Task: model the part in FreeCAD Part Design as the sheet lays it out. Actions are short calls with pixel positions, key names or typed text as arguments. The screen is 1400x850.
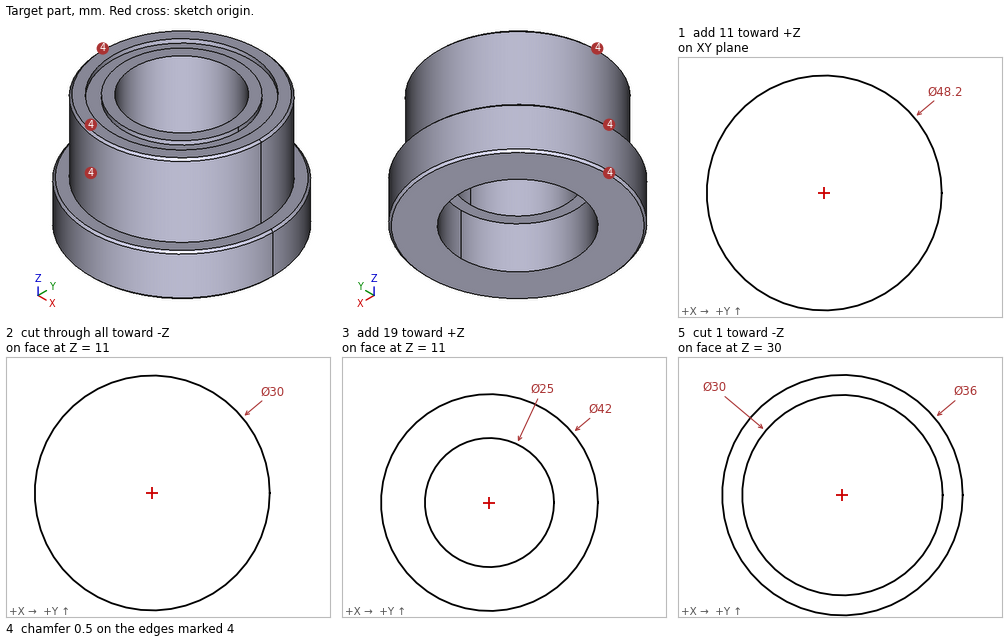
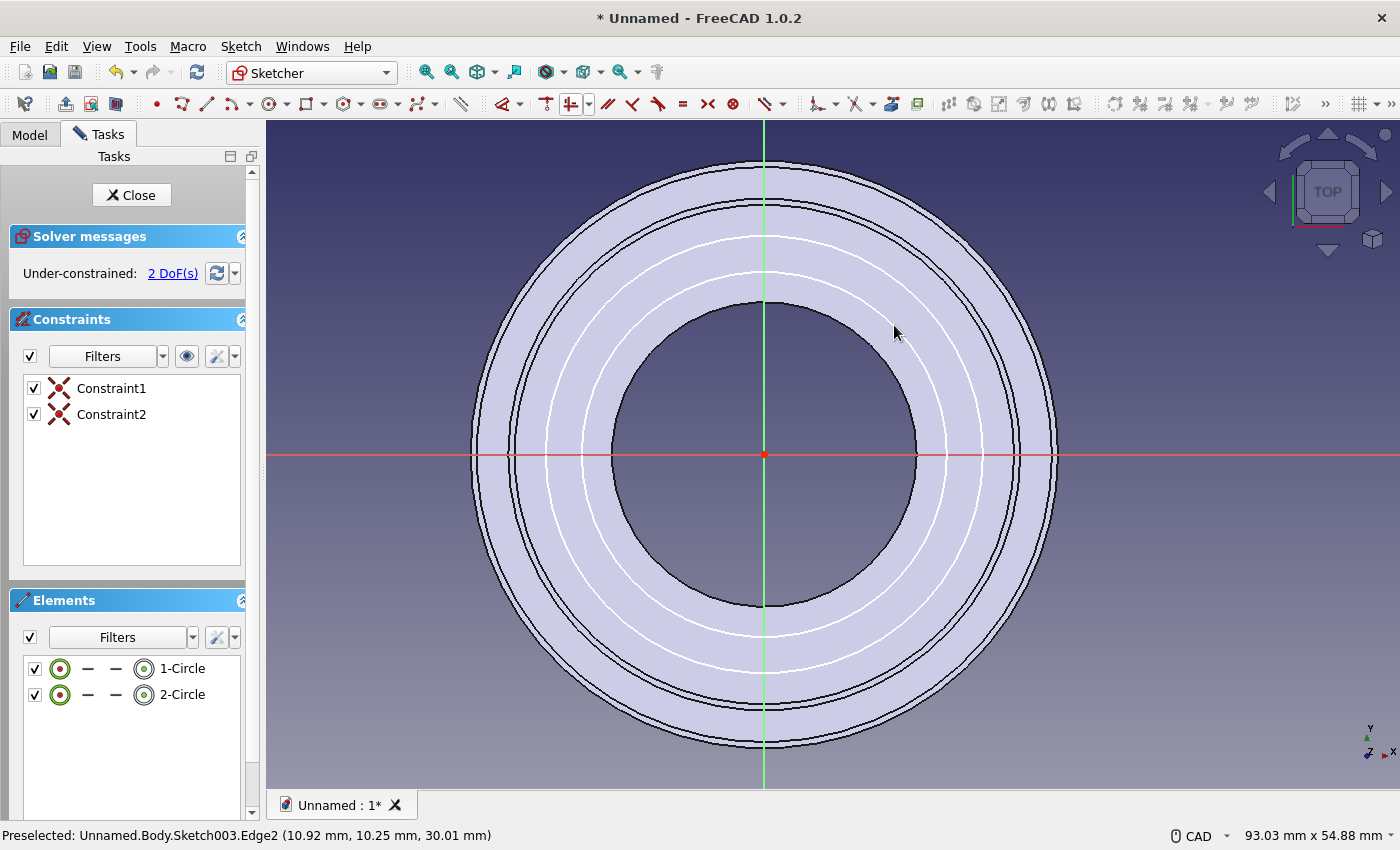
key(d)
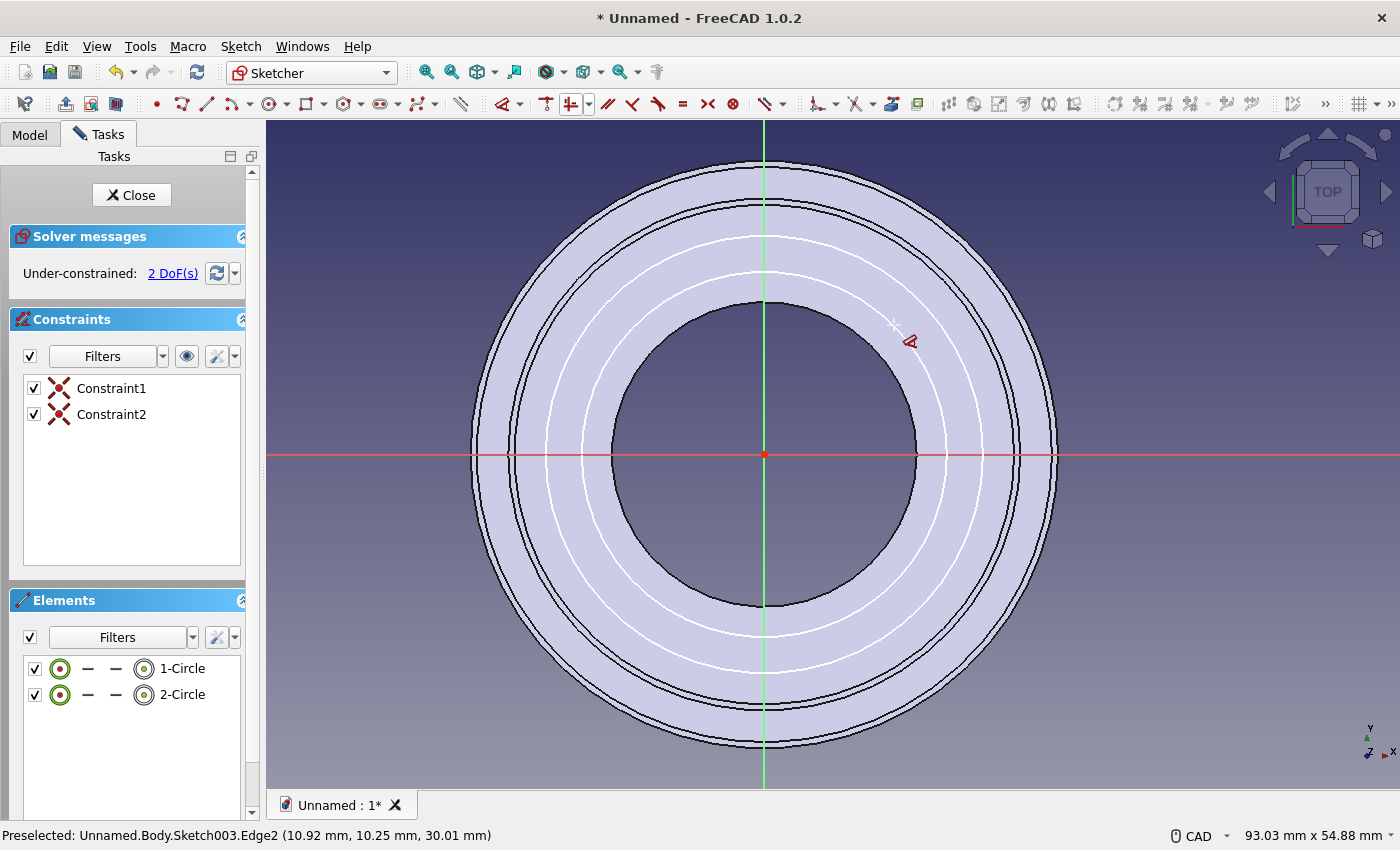
click(918, 299)
click(940, 276)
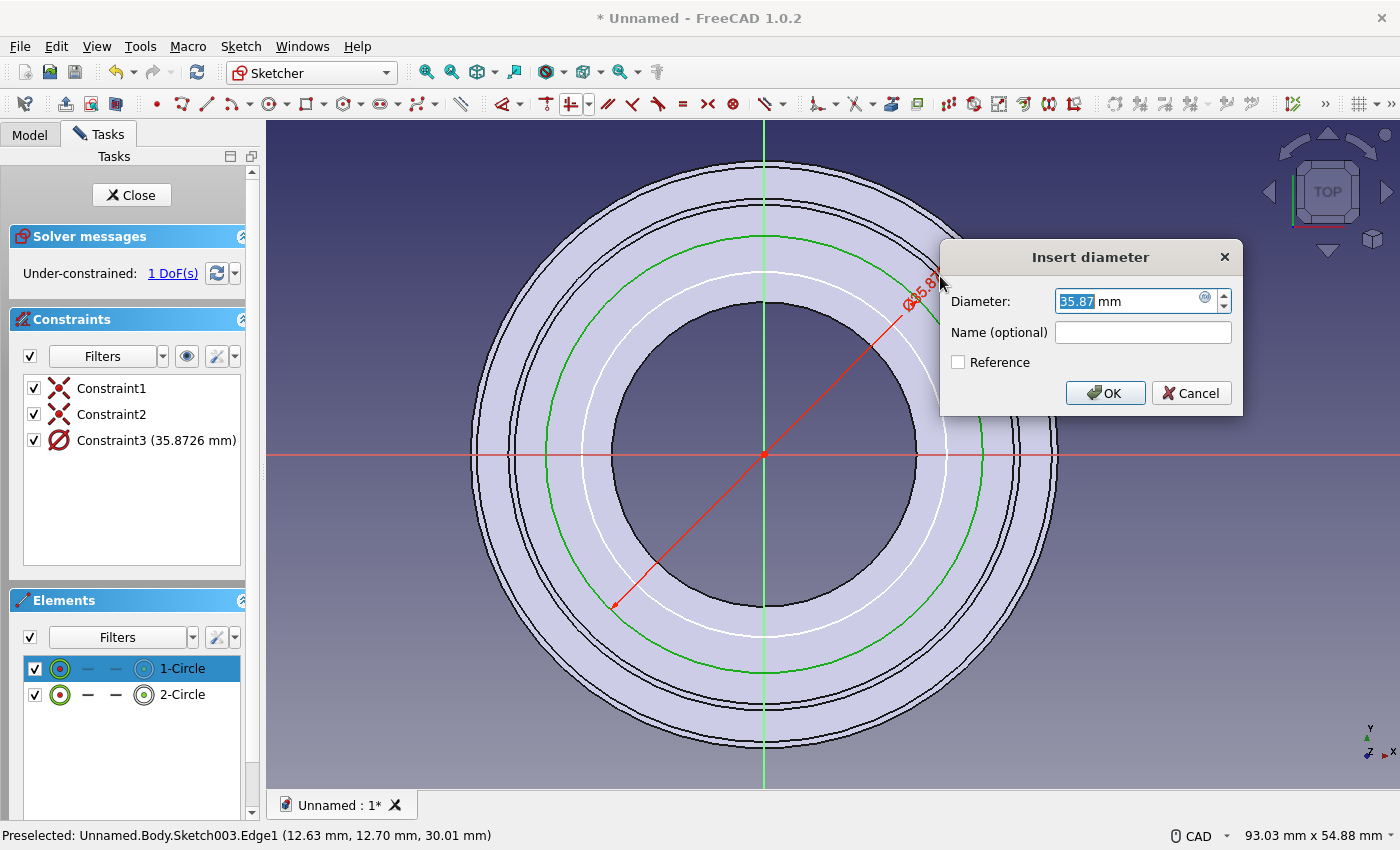
text(36)
key(Return)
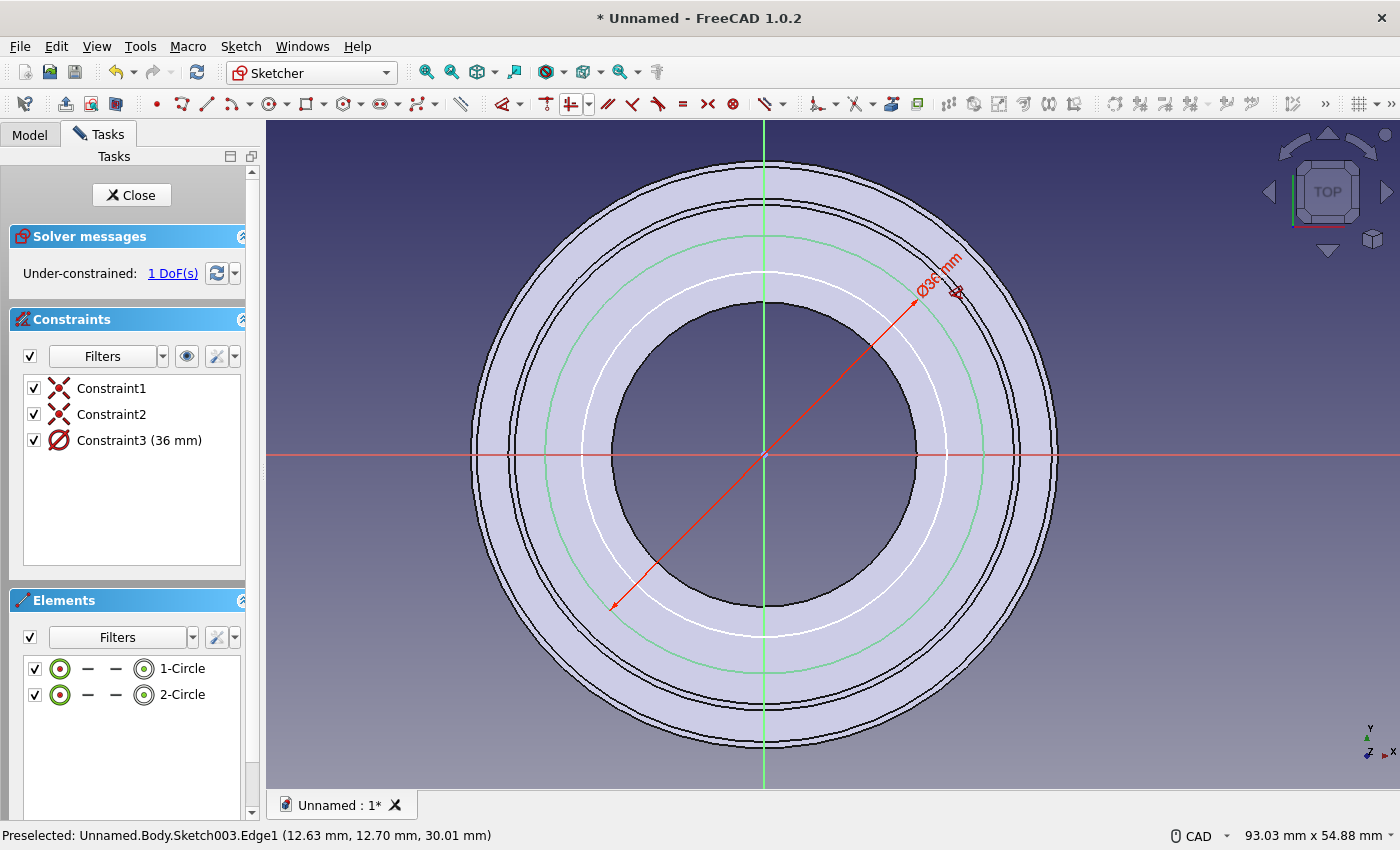
click(893, 325)
click(992, 387)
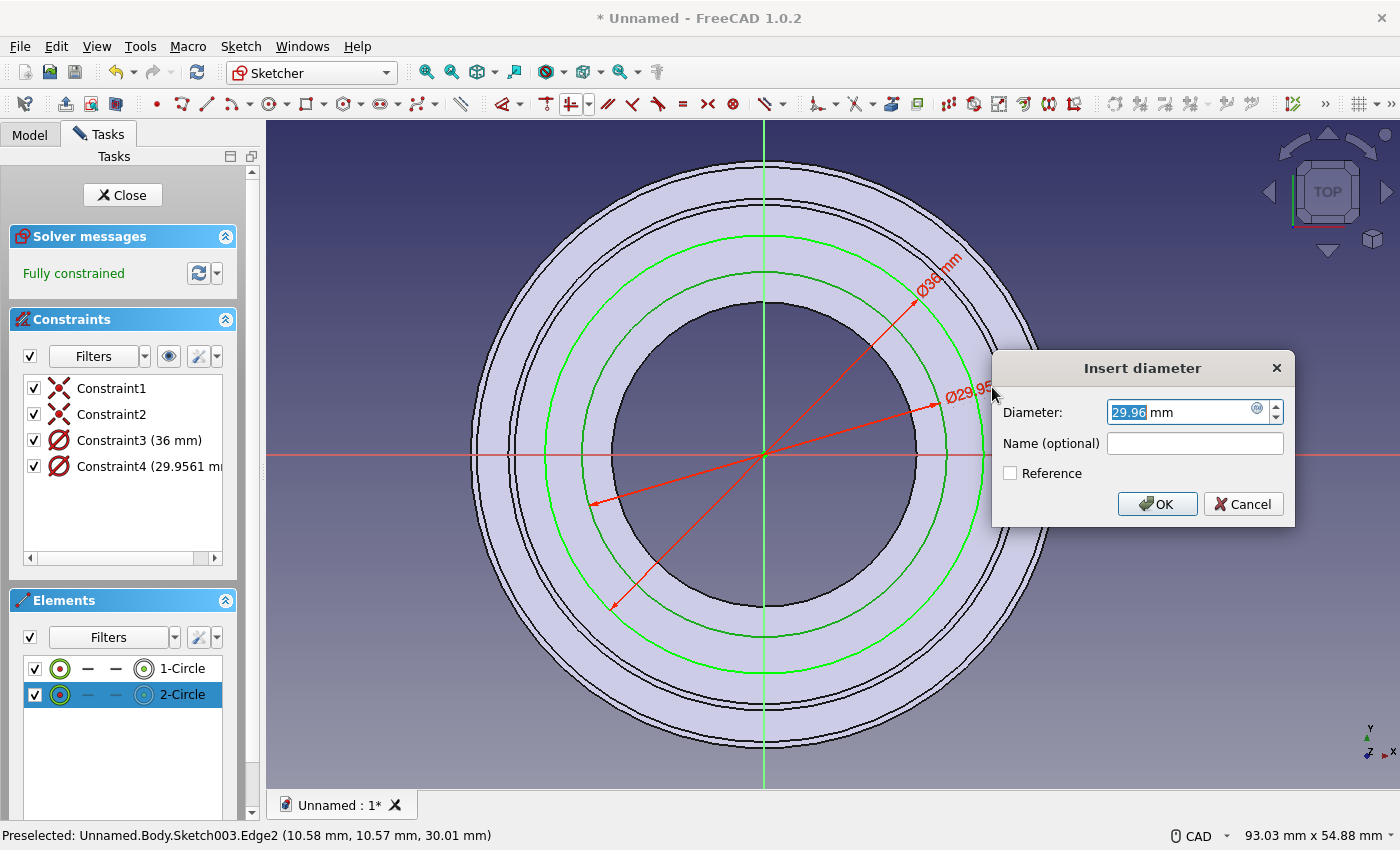
text(30)
key(Return)
key(Escape)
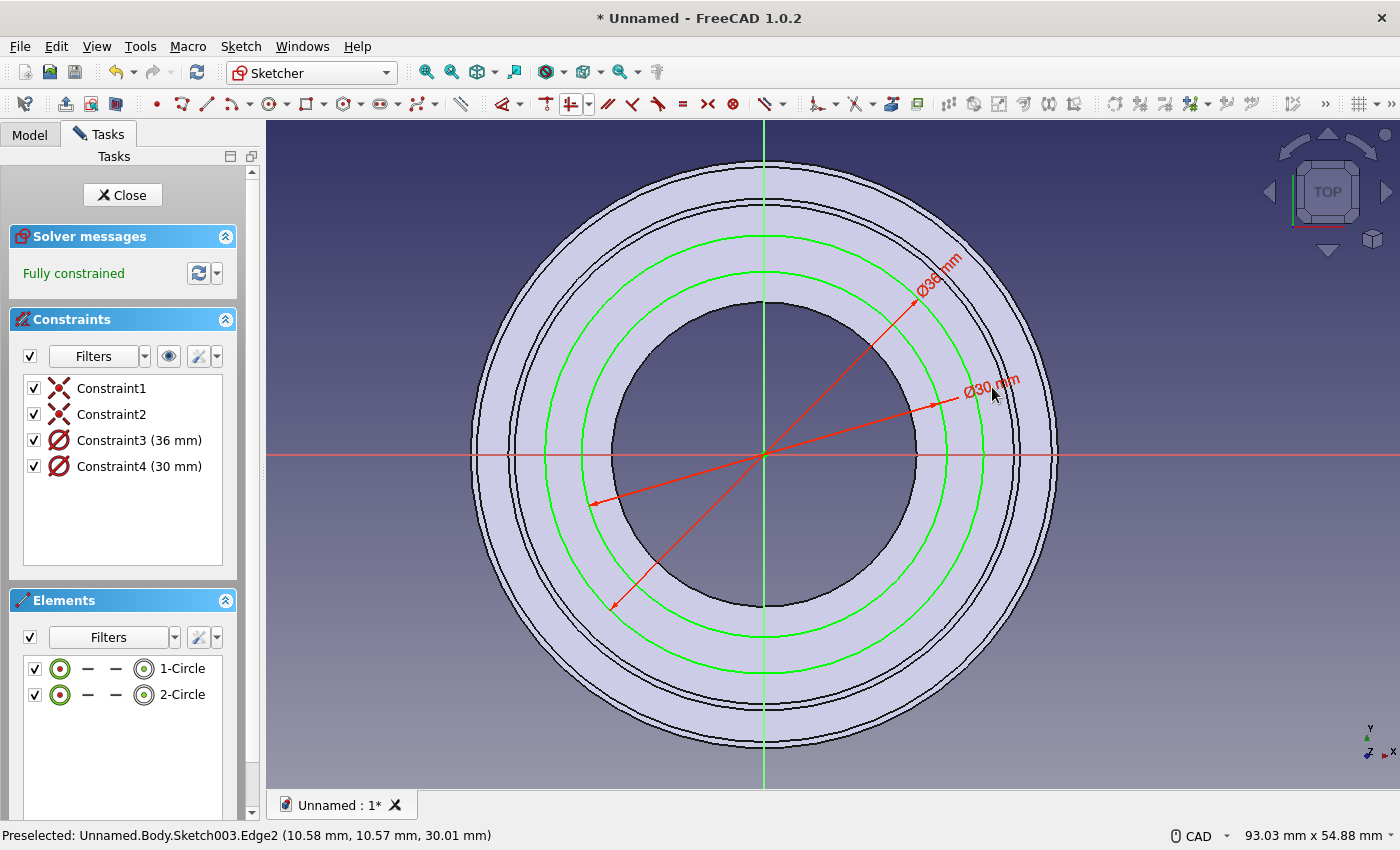
click(123, 195)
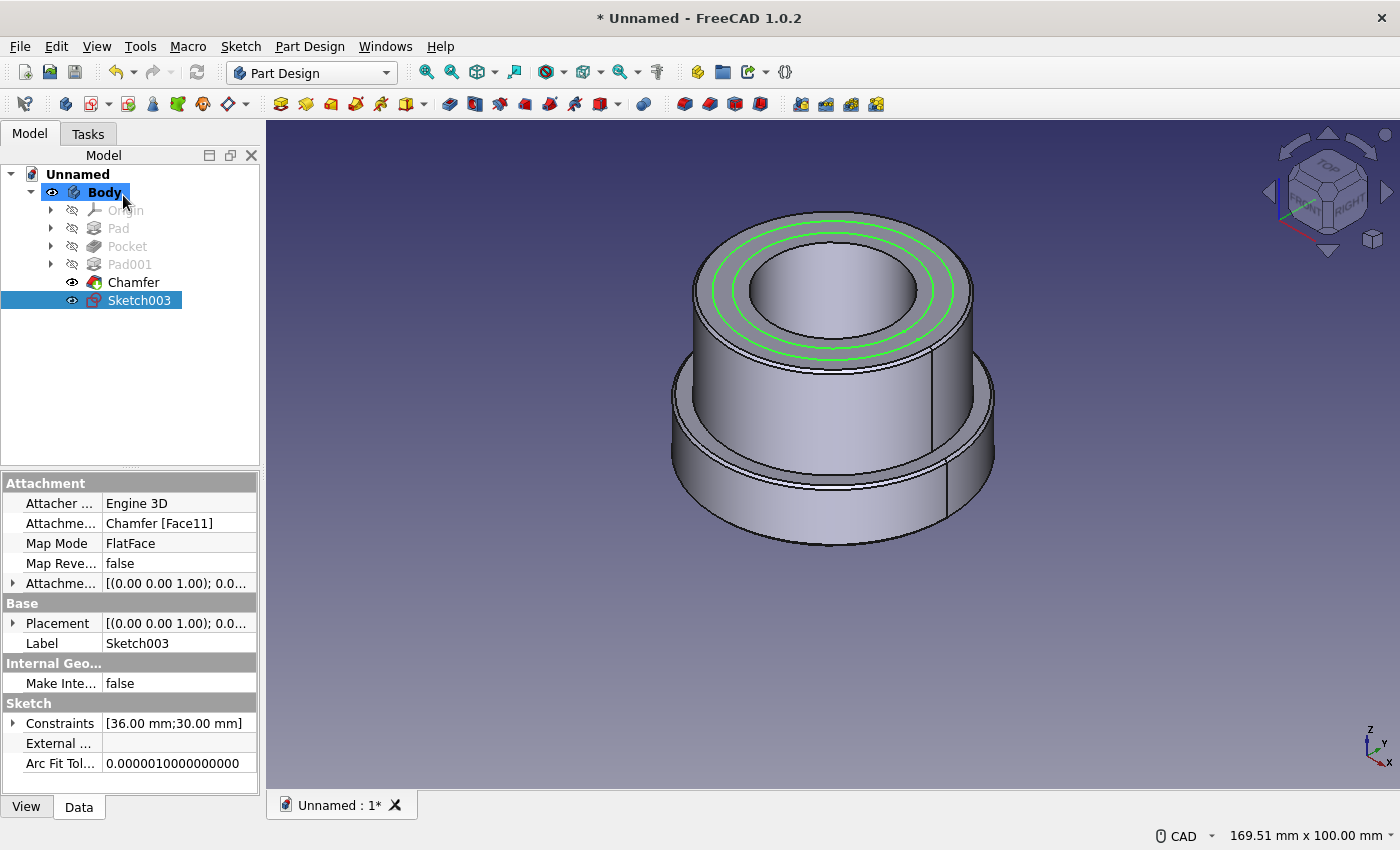
click(450, 104)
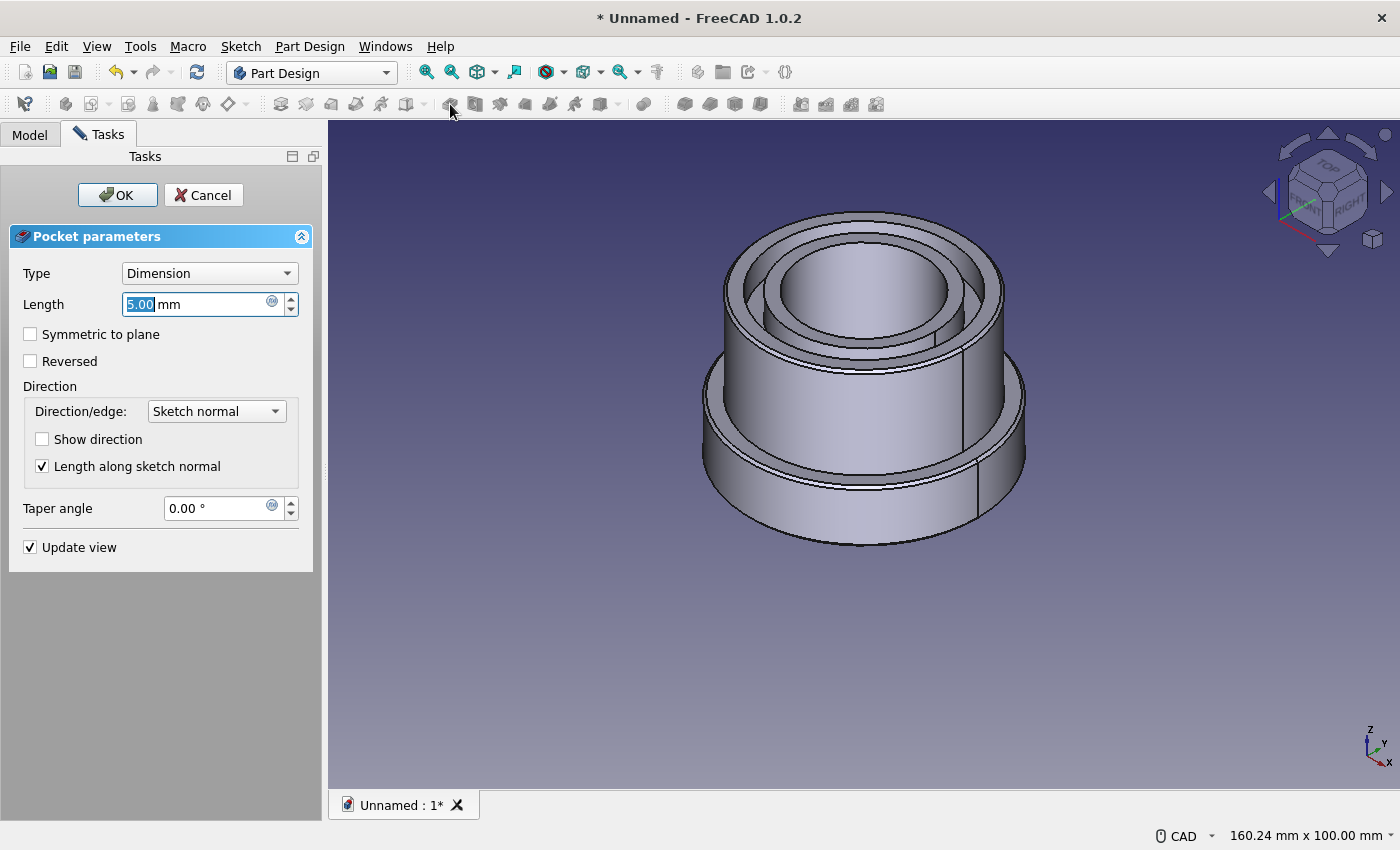
text(1)
key(Tab)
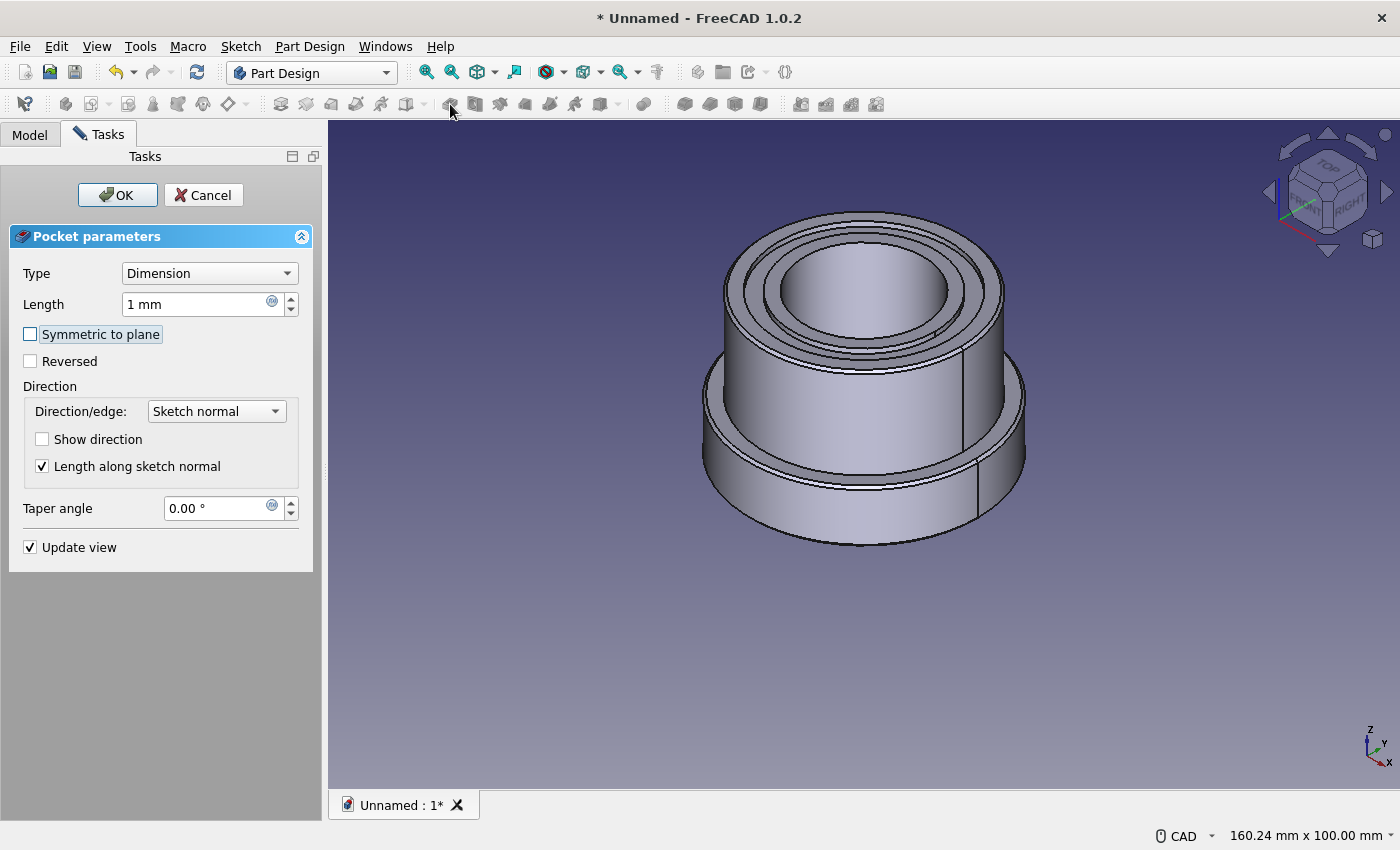
click(118, 195)